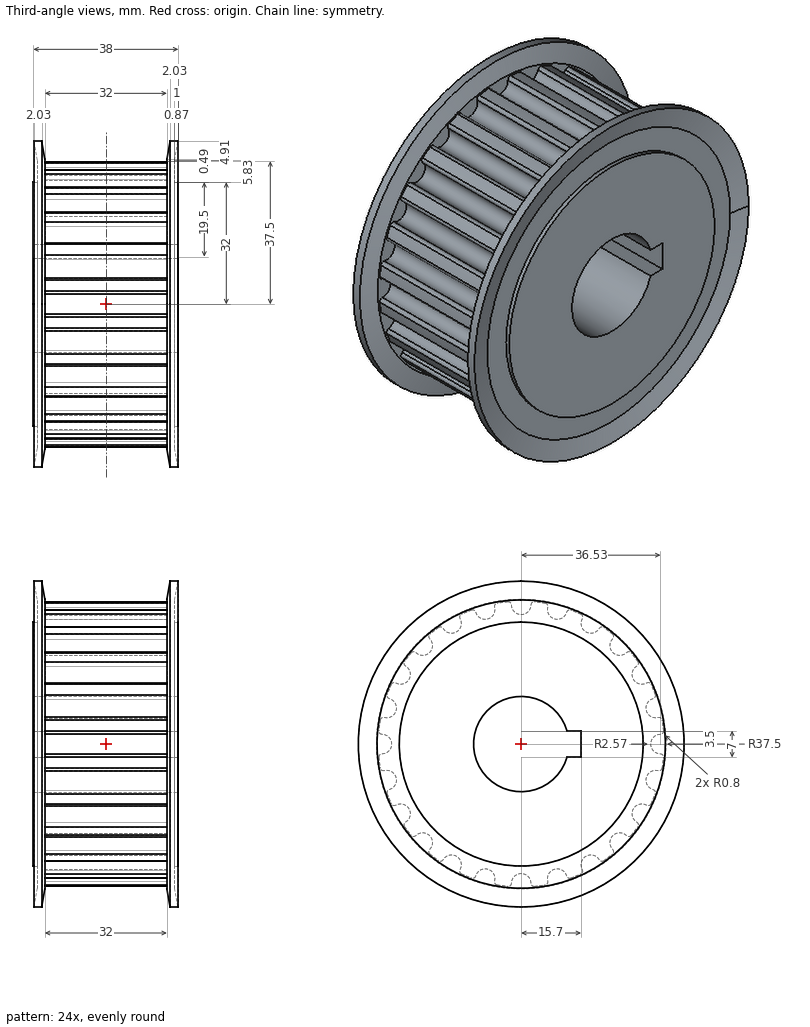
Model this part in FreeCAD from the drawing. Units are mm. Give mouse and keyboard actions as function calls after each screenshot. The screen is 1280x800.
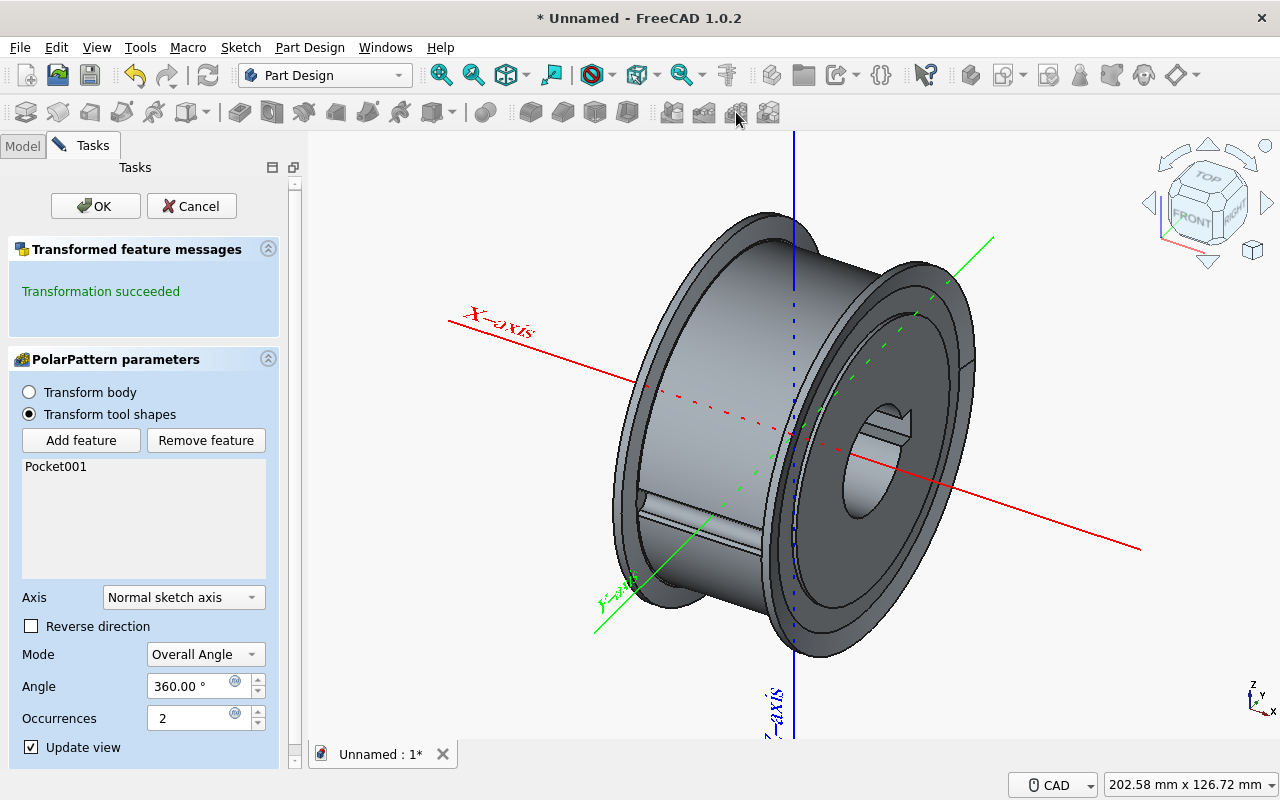
click(184, 598)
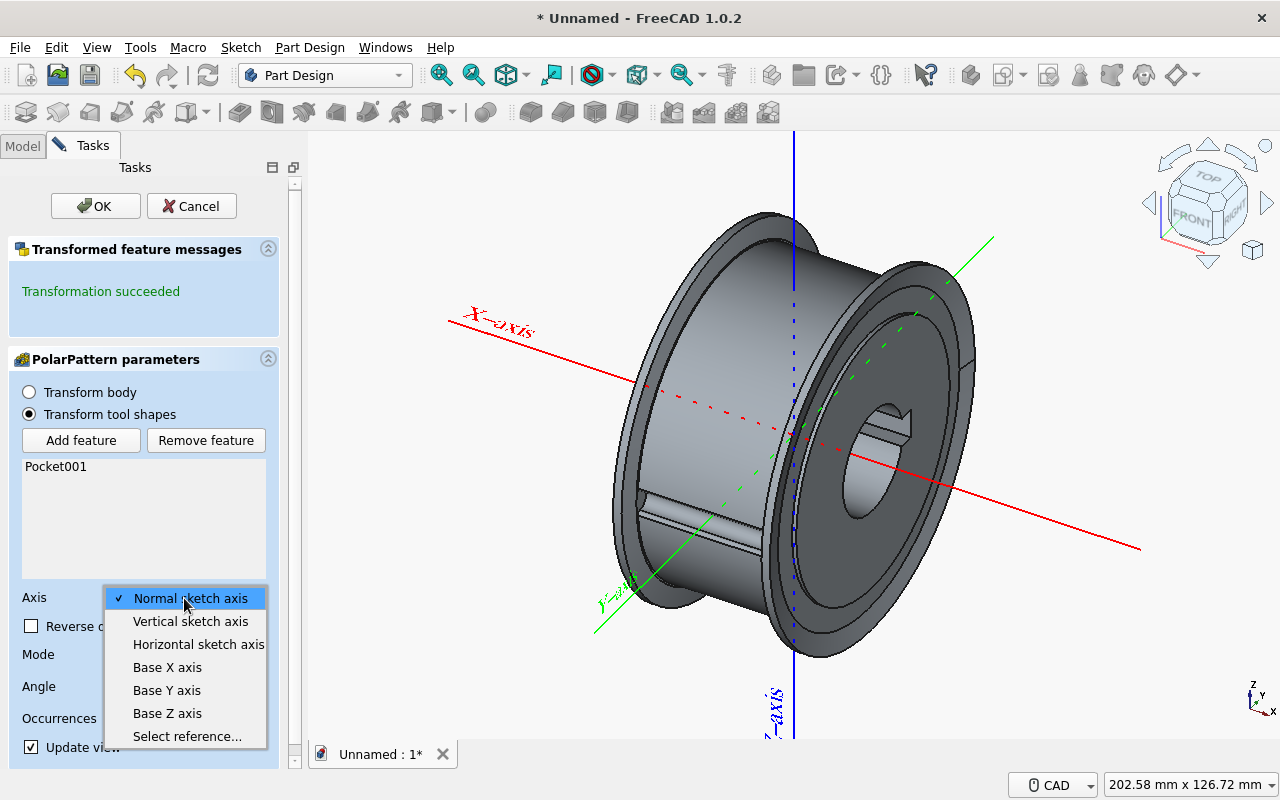
click(184, 668)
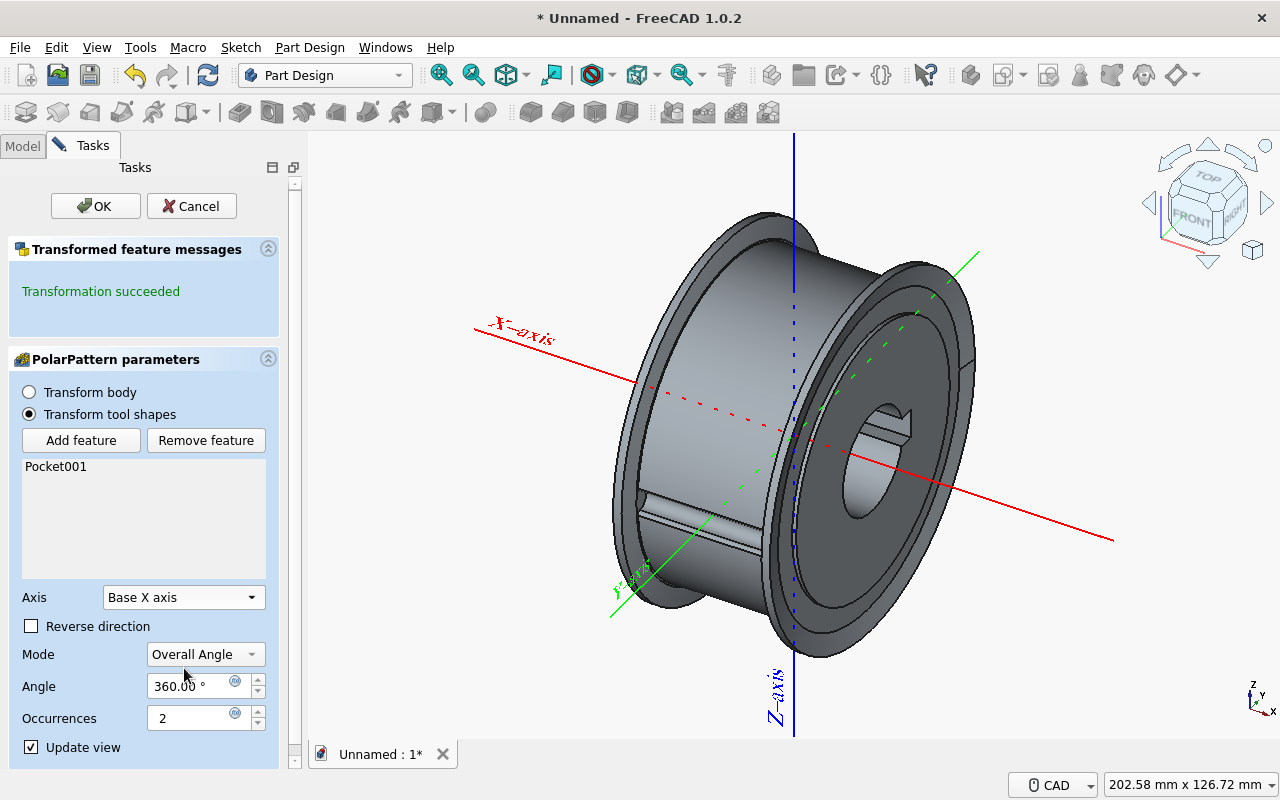
triple_click(198, 718)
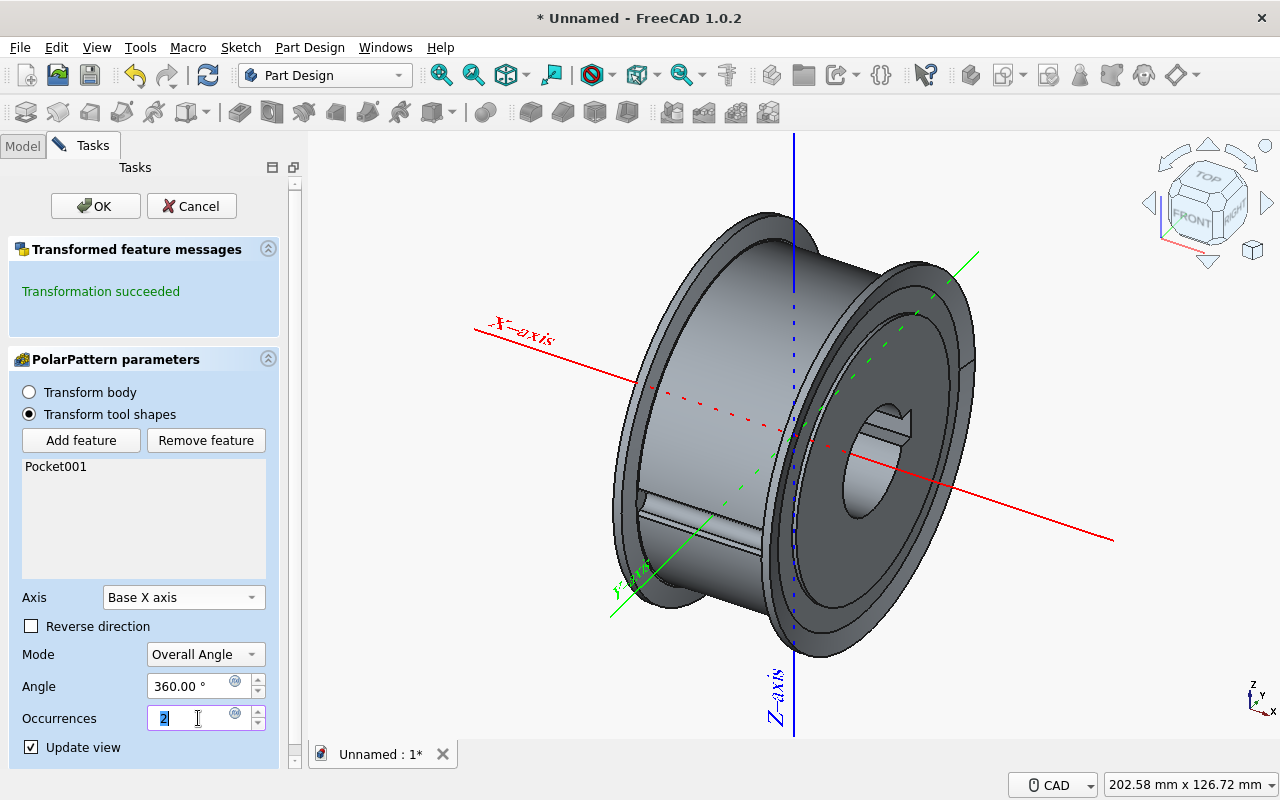
text(24)
key(Tab)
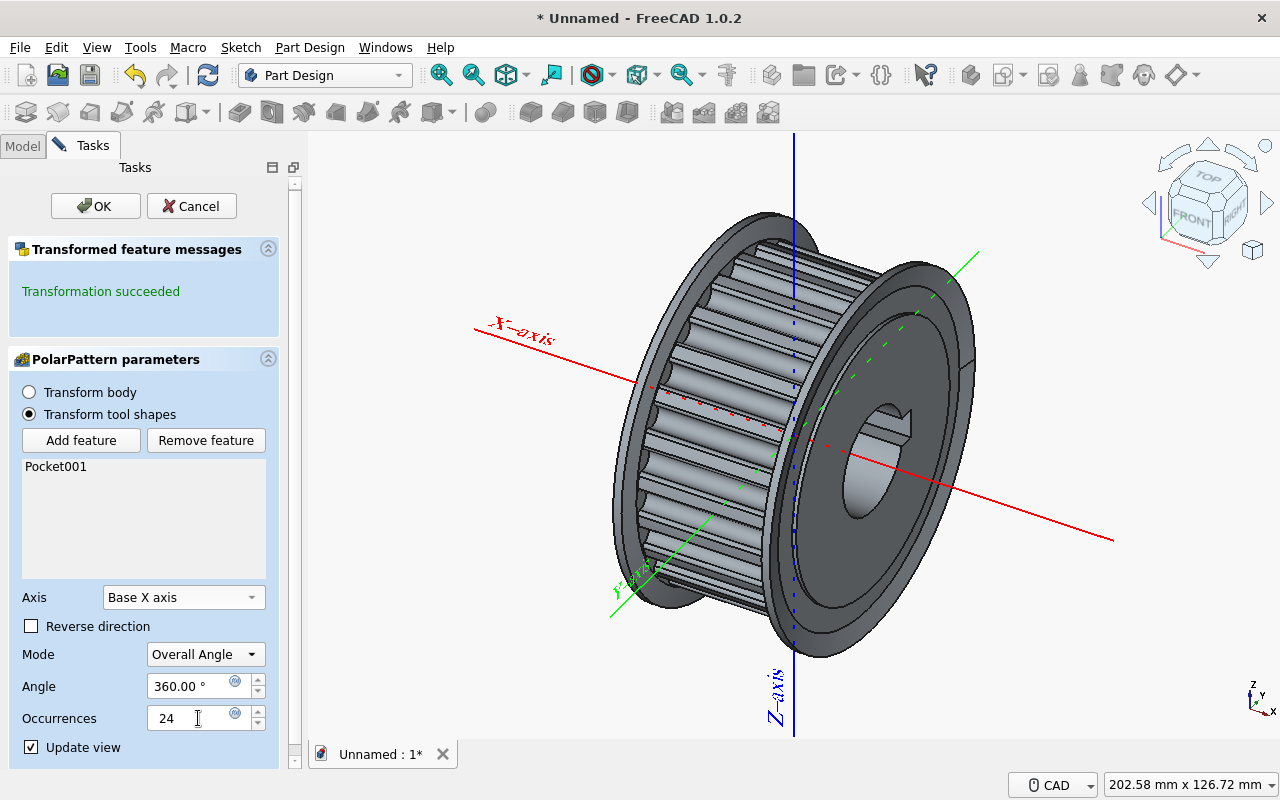
click(96, 206)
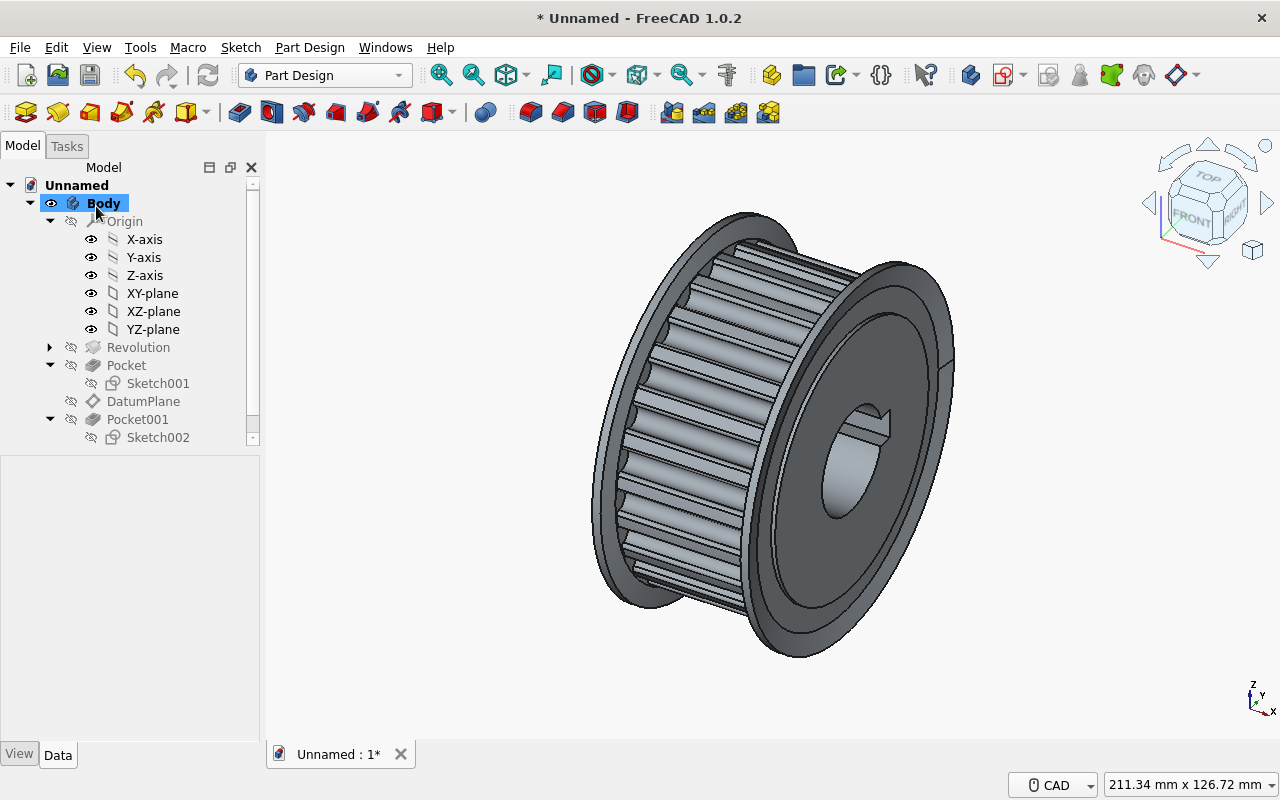
key(0)